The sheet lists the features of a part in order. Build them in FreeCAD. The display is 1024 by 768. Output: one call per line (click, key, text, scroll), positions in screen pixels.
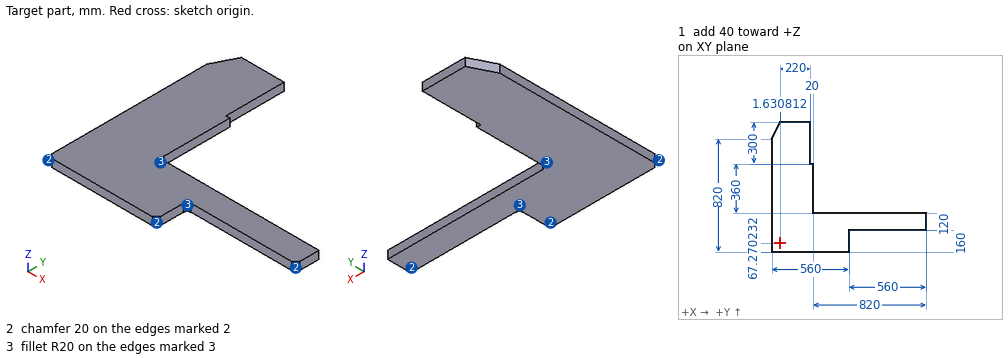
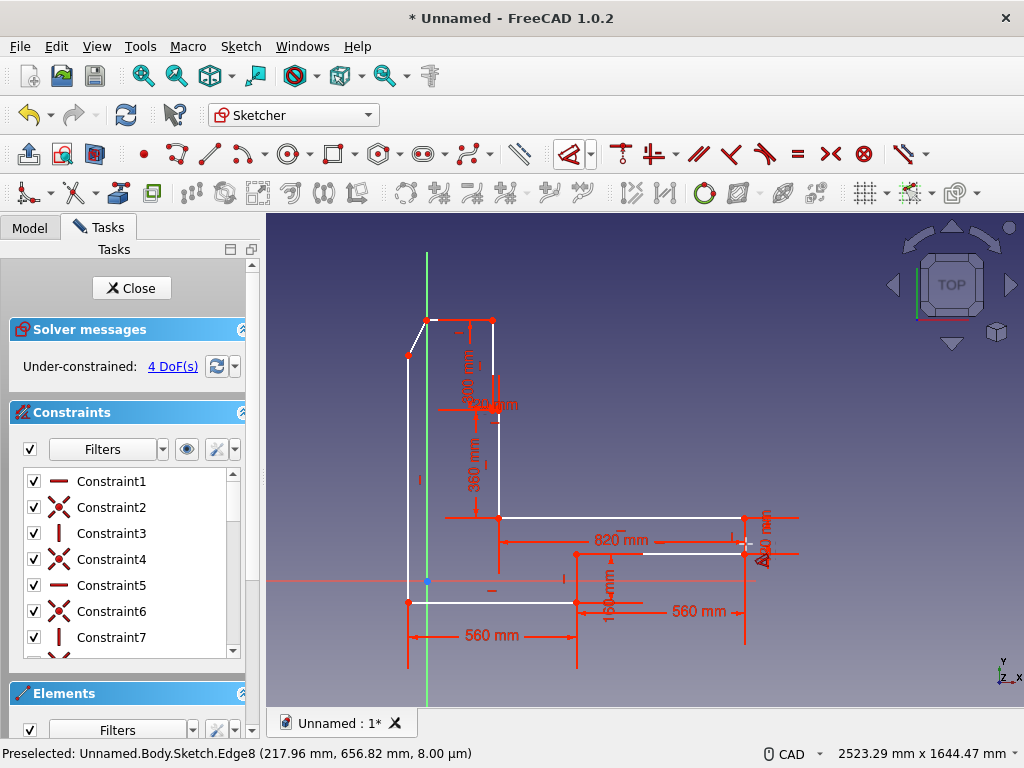
click(473, 320)
click(460, 286)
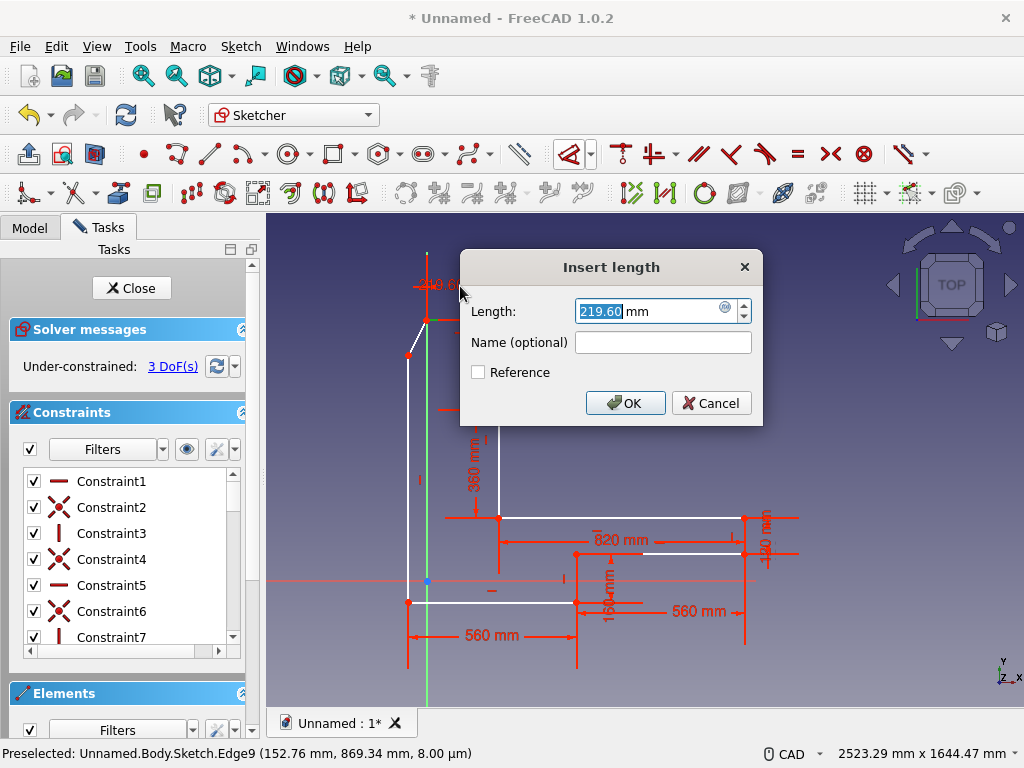
text(220)
key(Return)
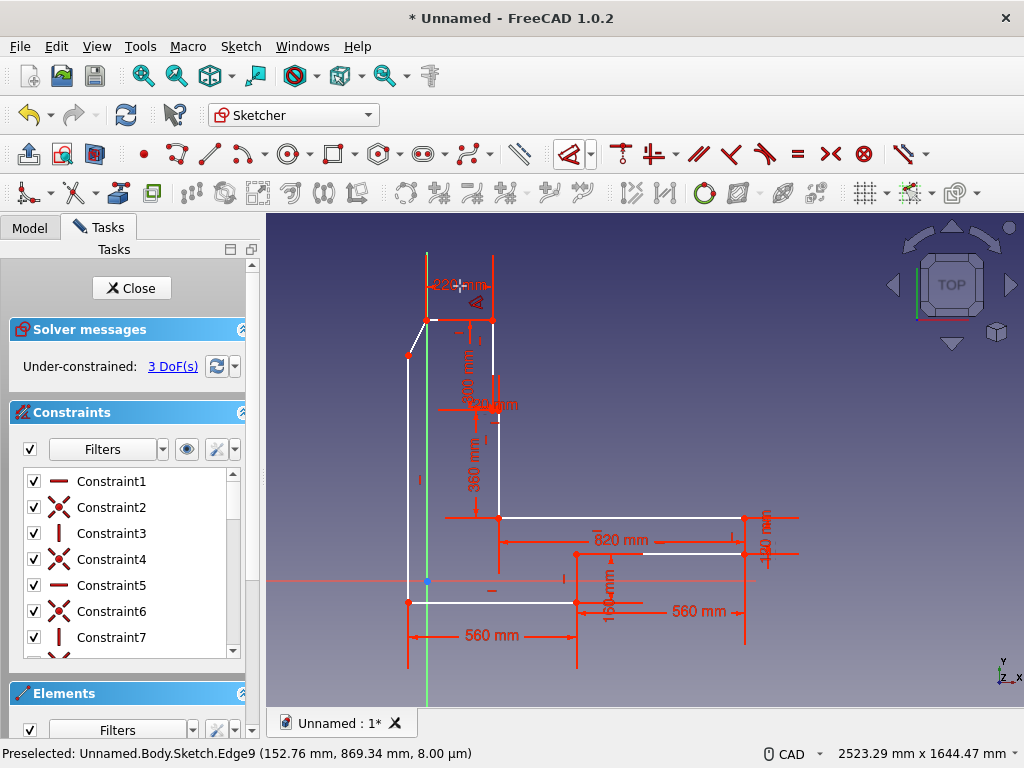
click(408, 430)
click(374, 479)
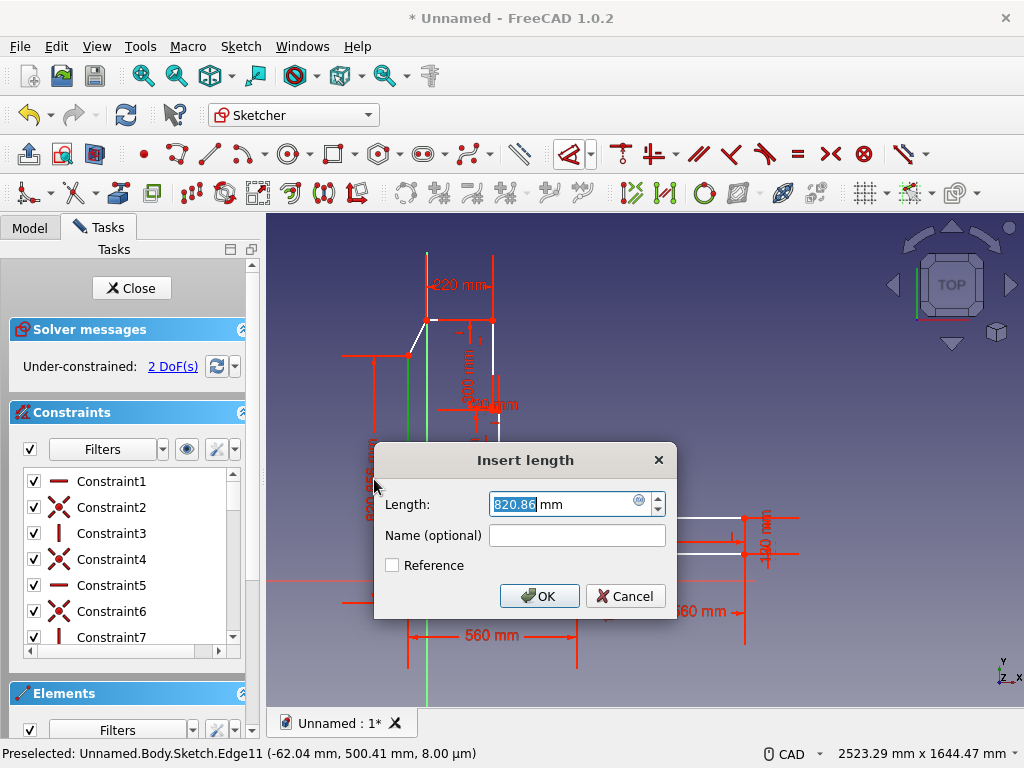
text(820)
key(Return)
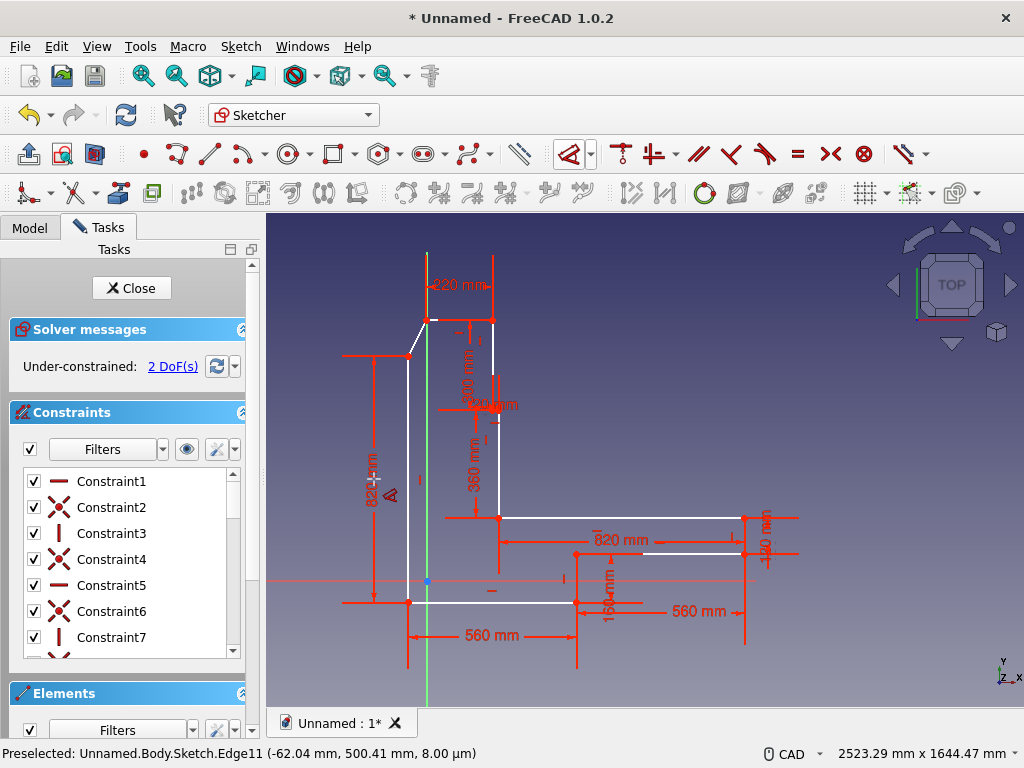
scroll(426, 320, up, 22)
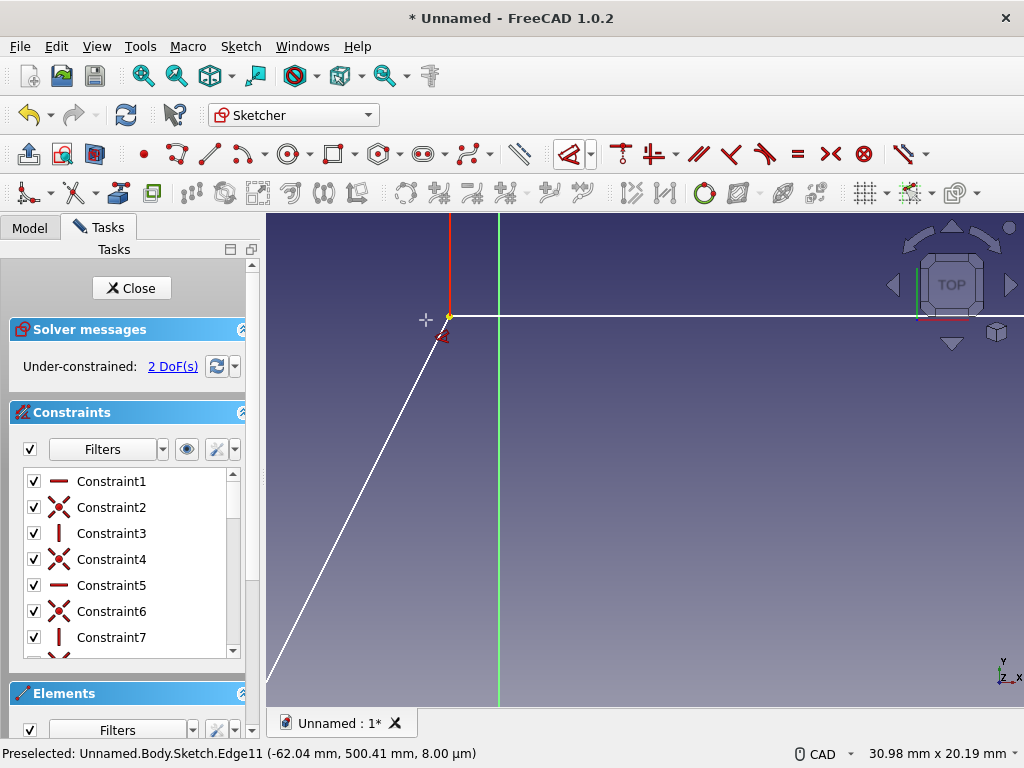
click(450, 316)
click(475, 282)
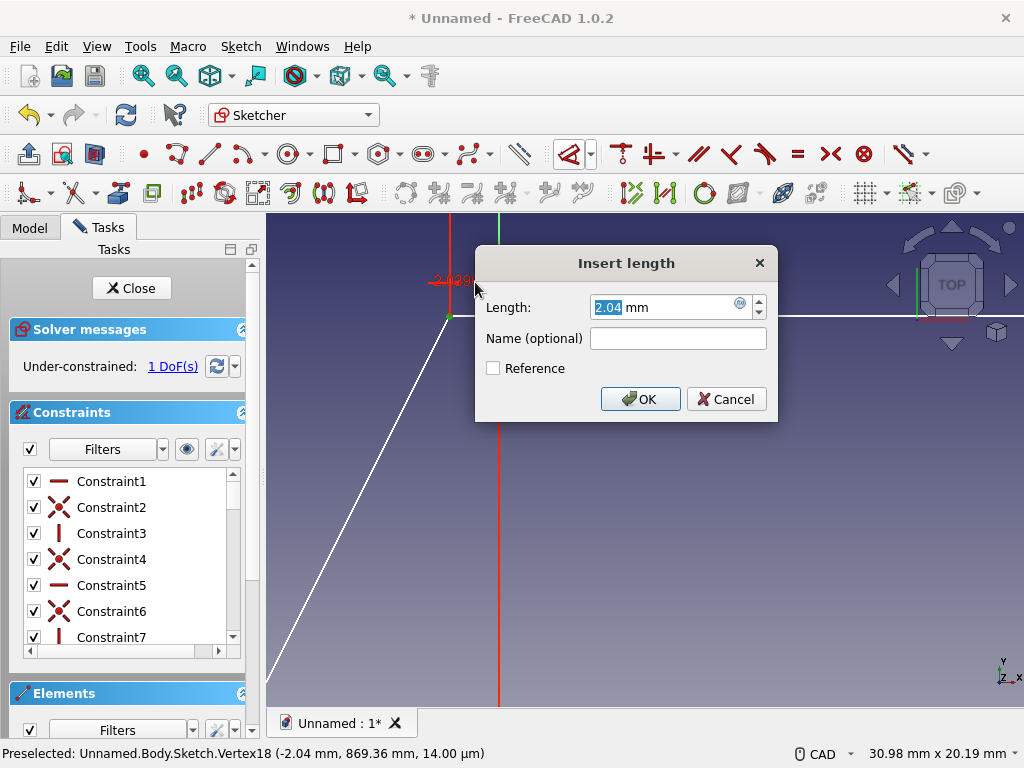
text(1.630812)
key(Return)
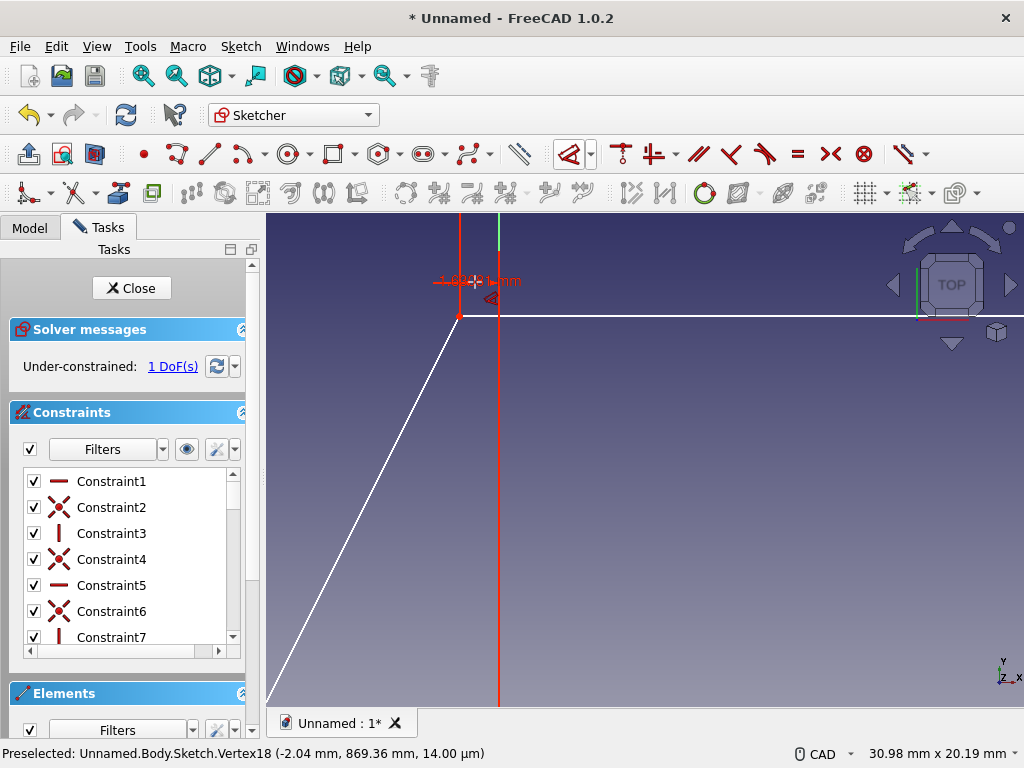
scroll(576, 460, down, 15)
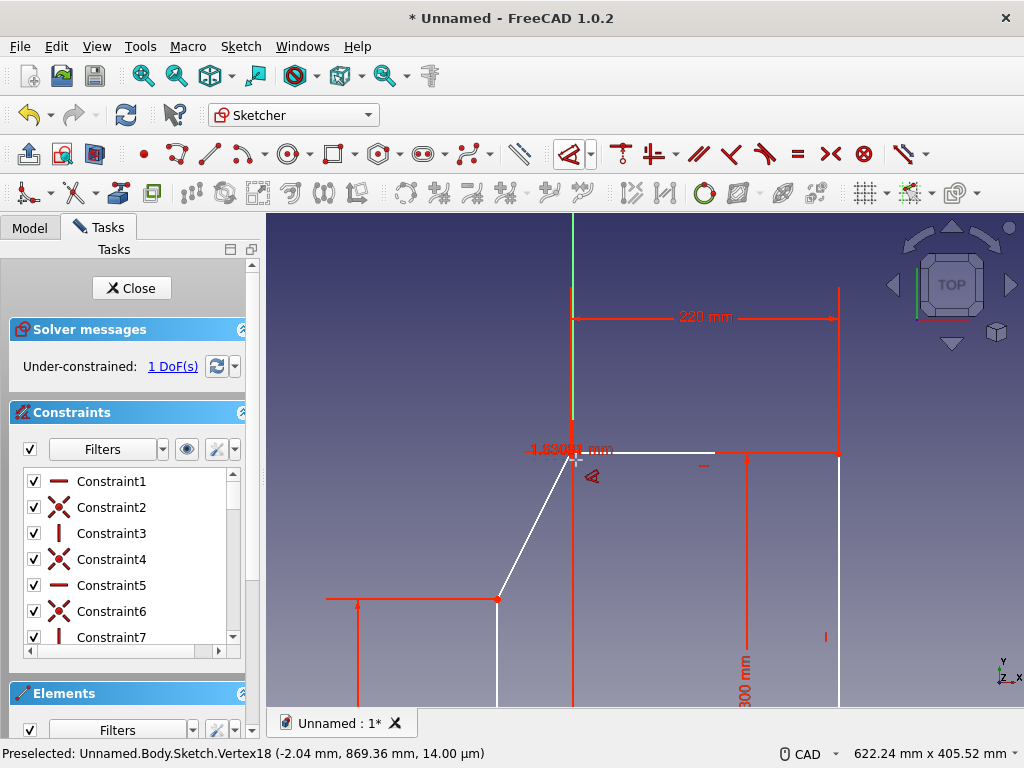
scroll(379, 276, down, 7)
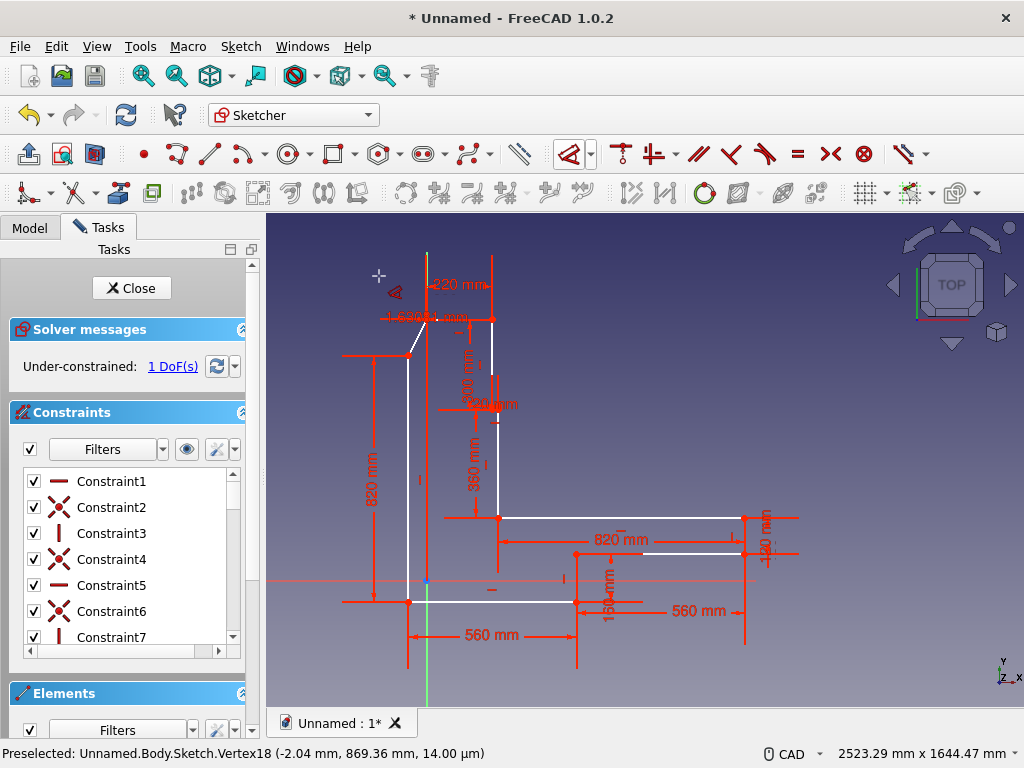
scroll(408, 602, up, 4)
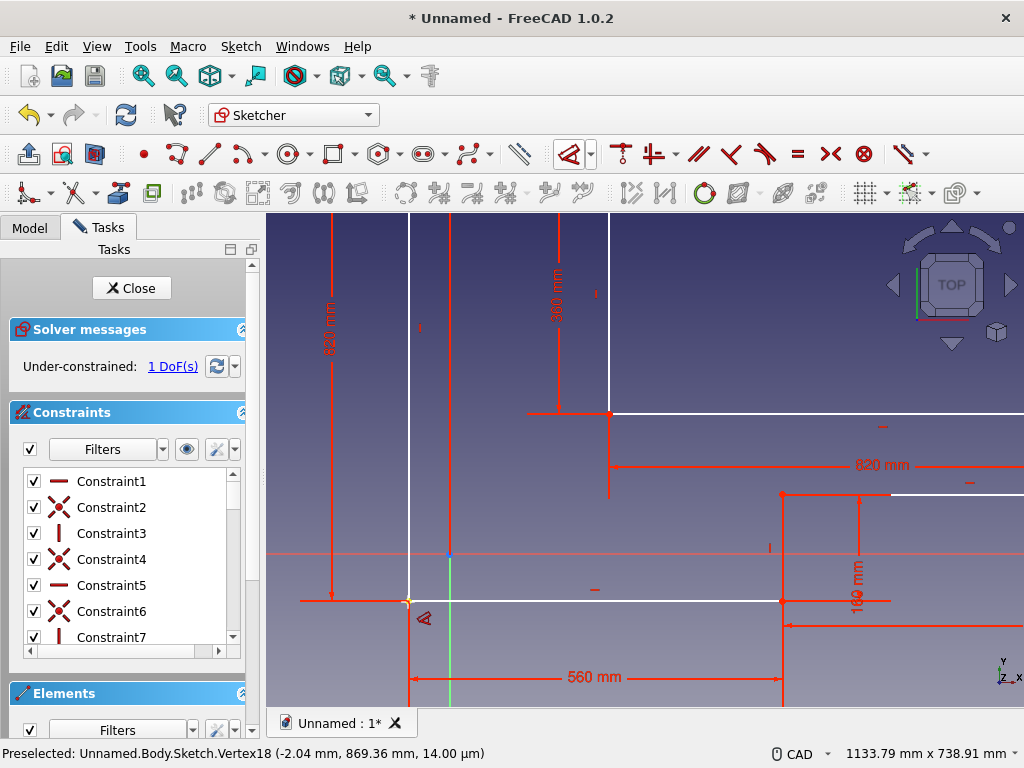
click(409, 601)
click(375, 578)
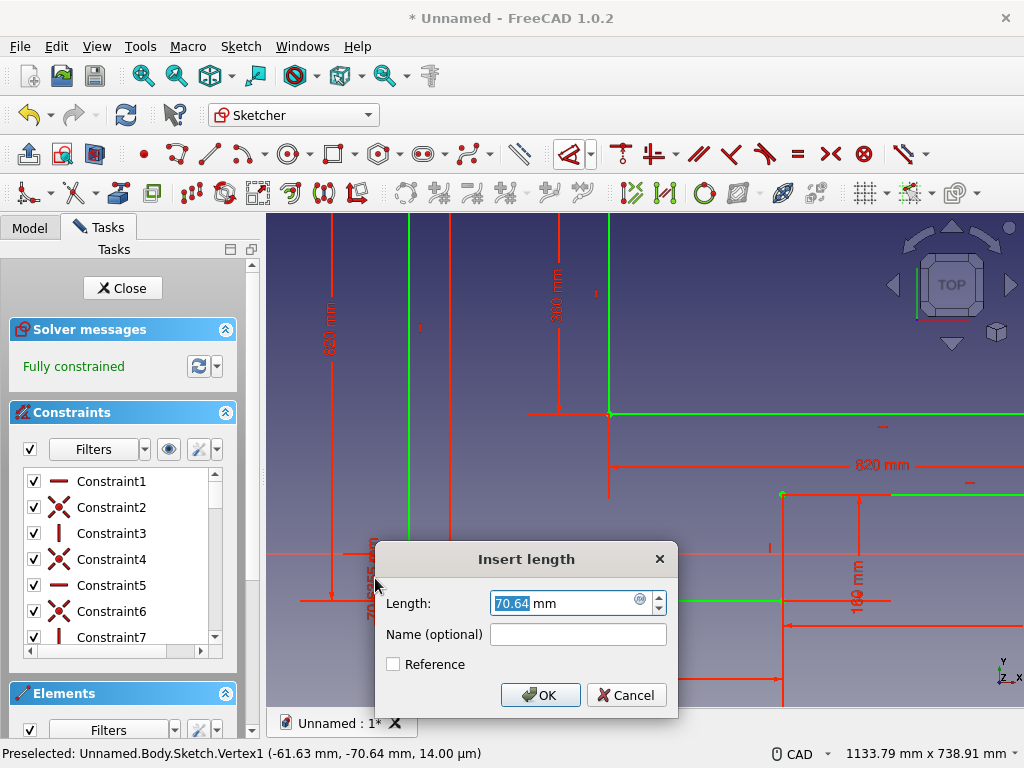
text(67.270232)
key(Return)
key(Escape)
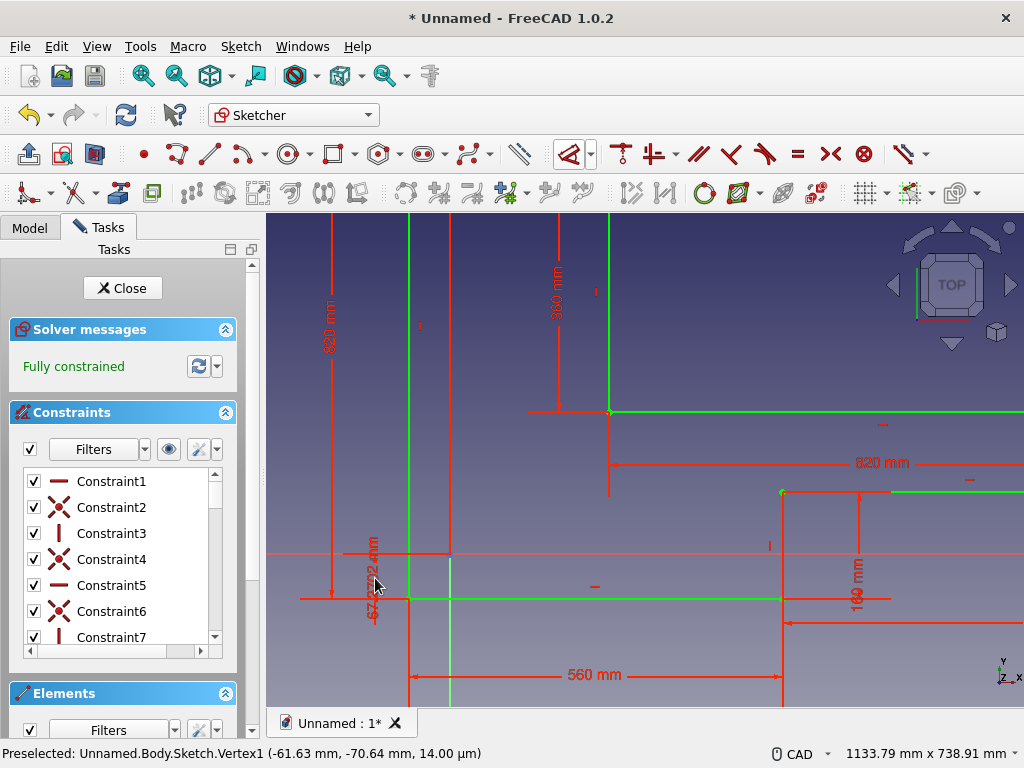
click(123, 288)